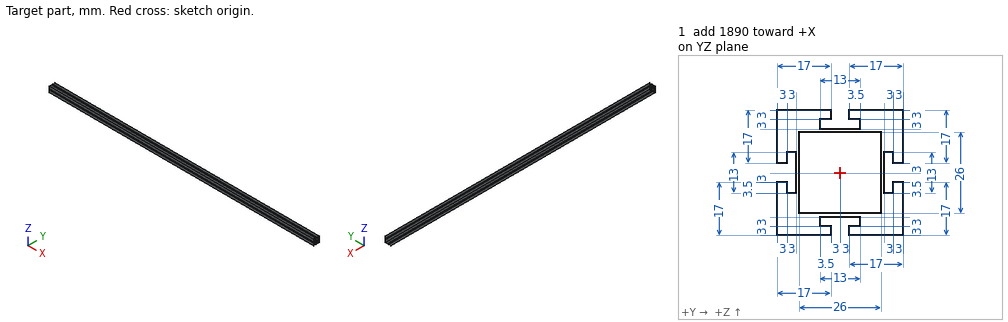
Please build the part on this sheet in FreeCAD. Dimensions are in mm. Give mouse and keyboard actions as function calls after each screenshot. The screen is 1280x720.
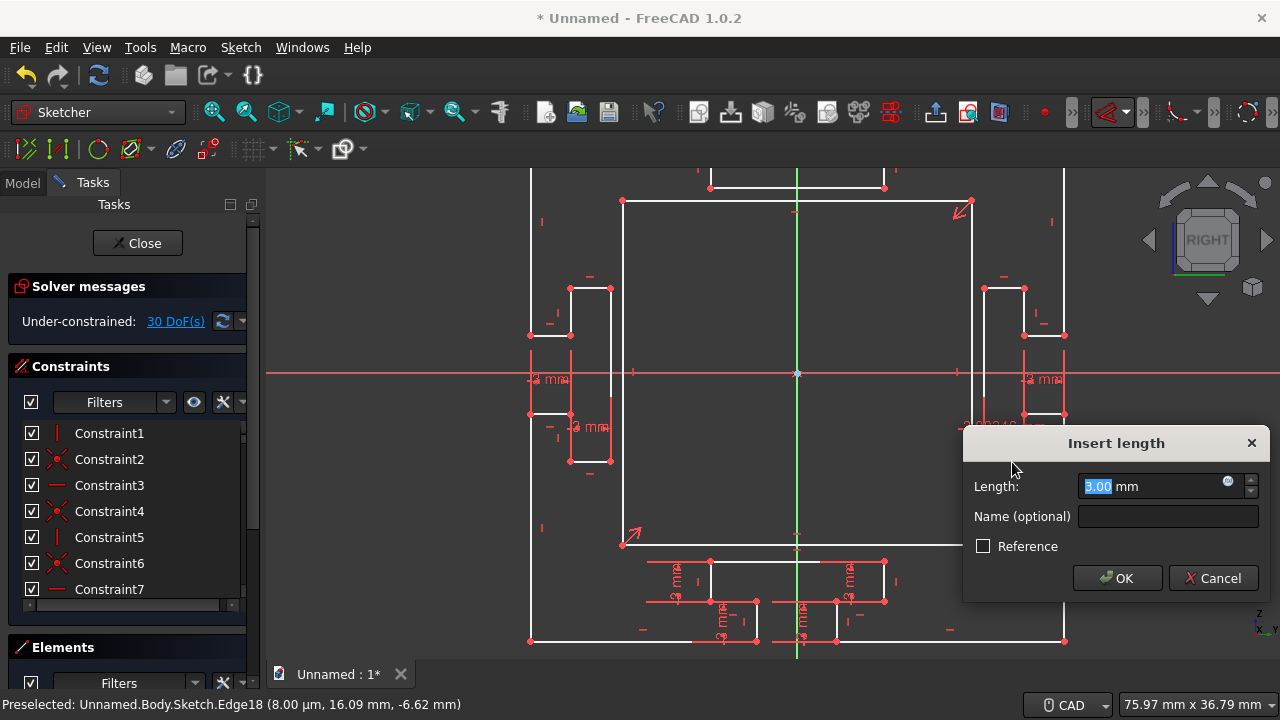
text(3)
key(Return)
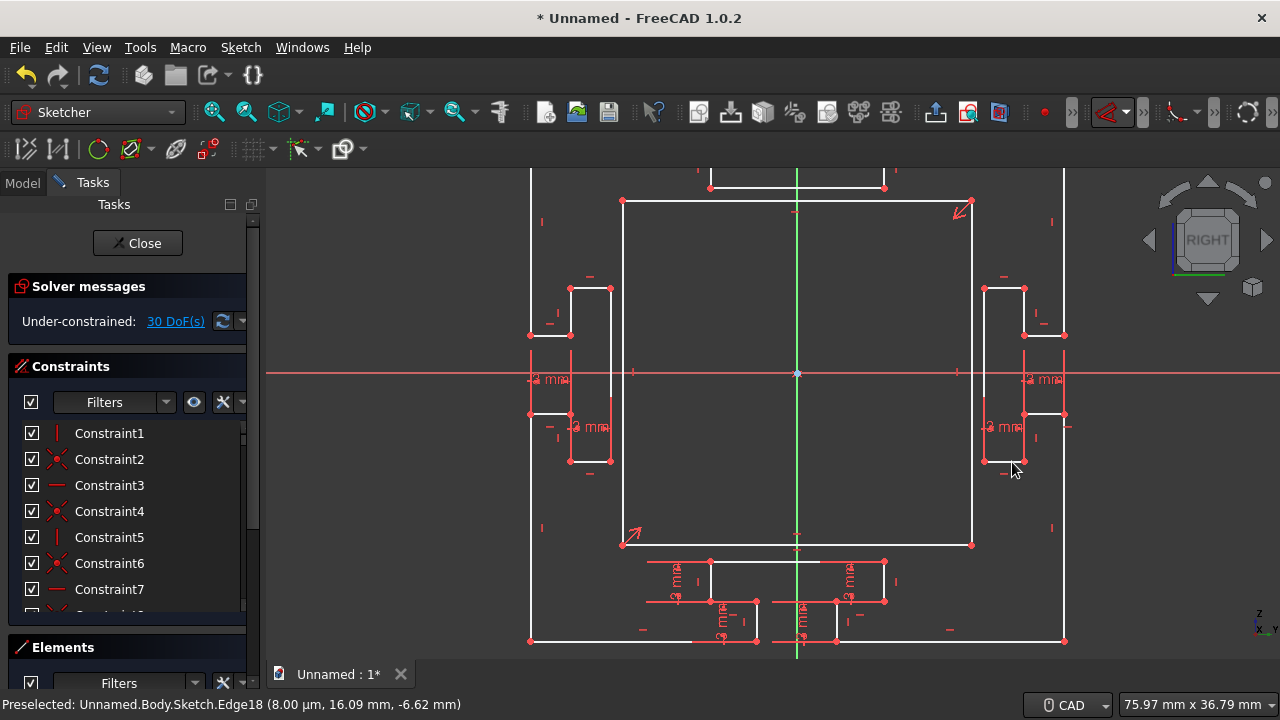
click(996, 288)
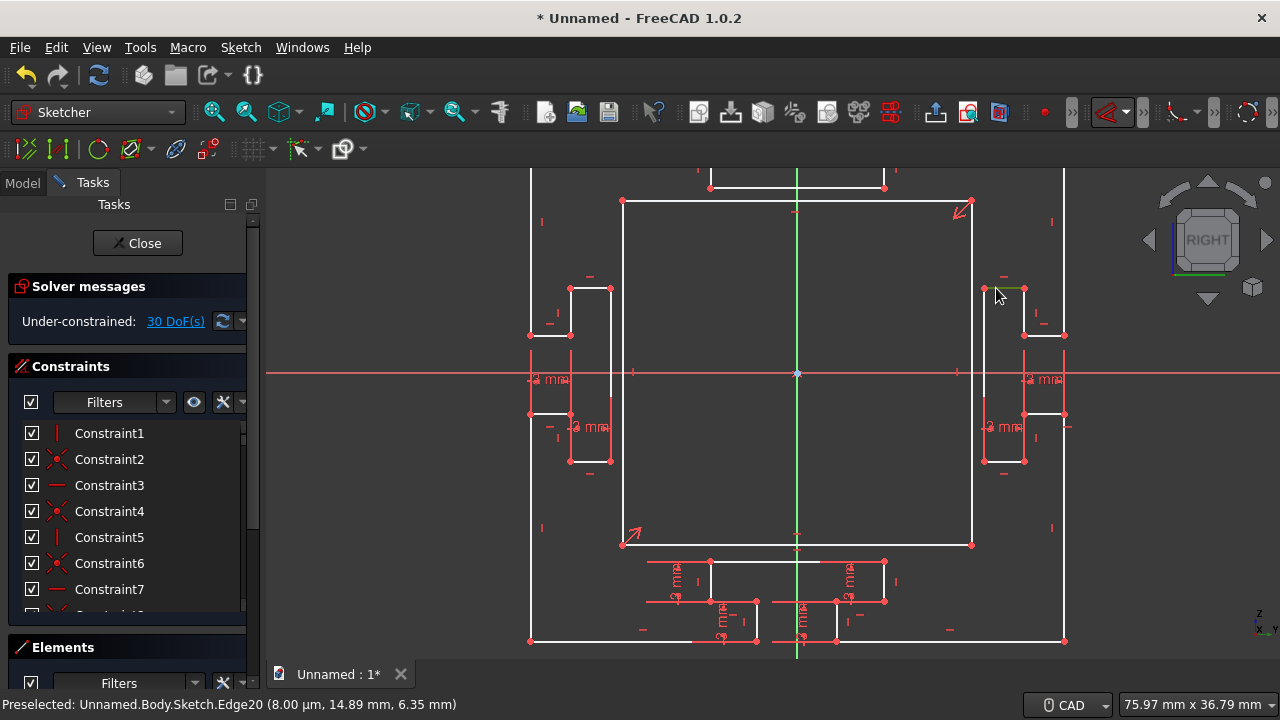
key(l)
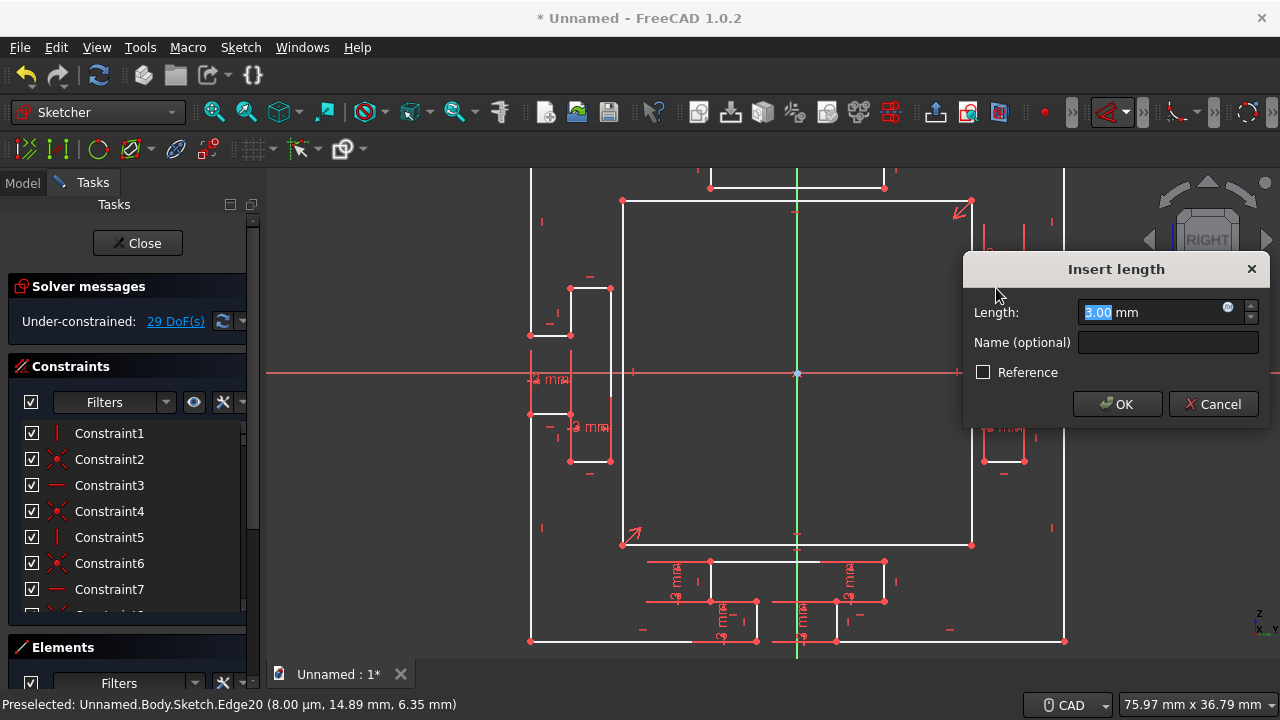
text(3)
key(Return)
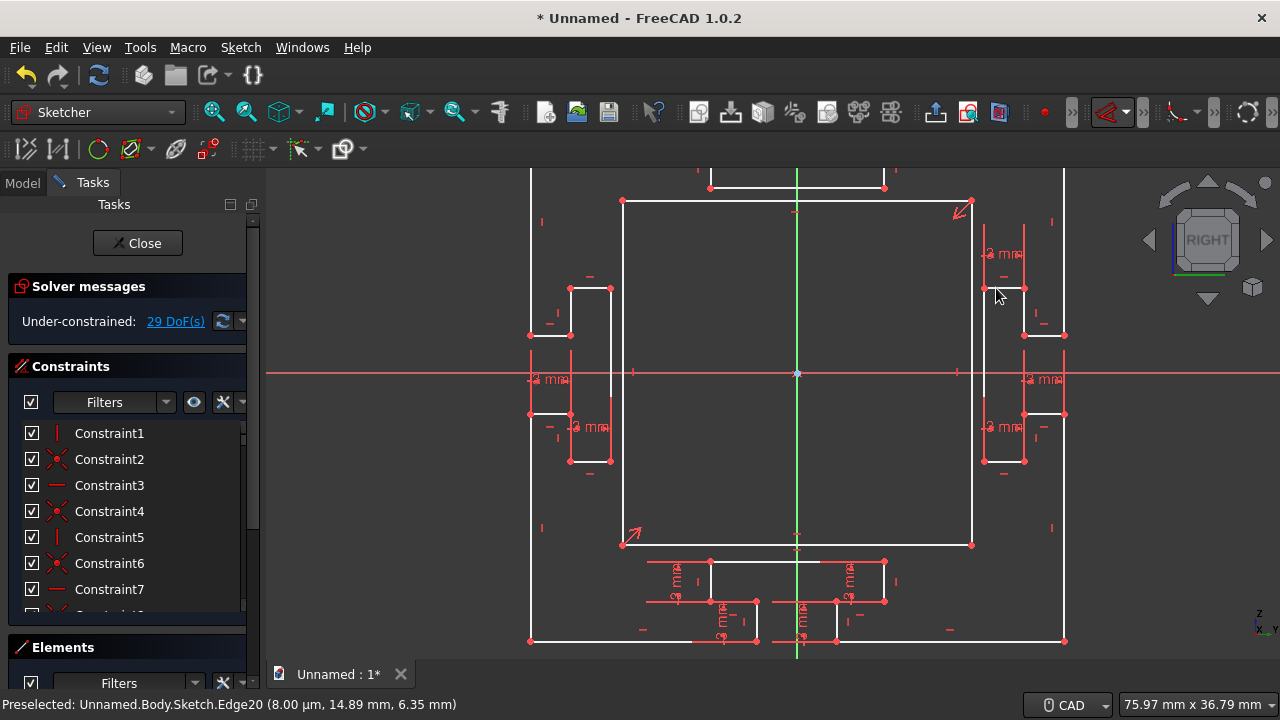
click(1036, 336)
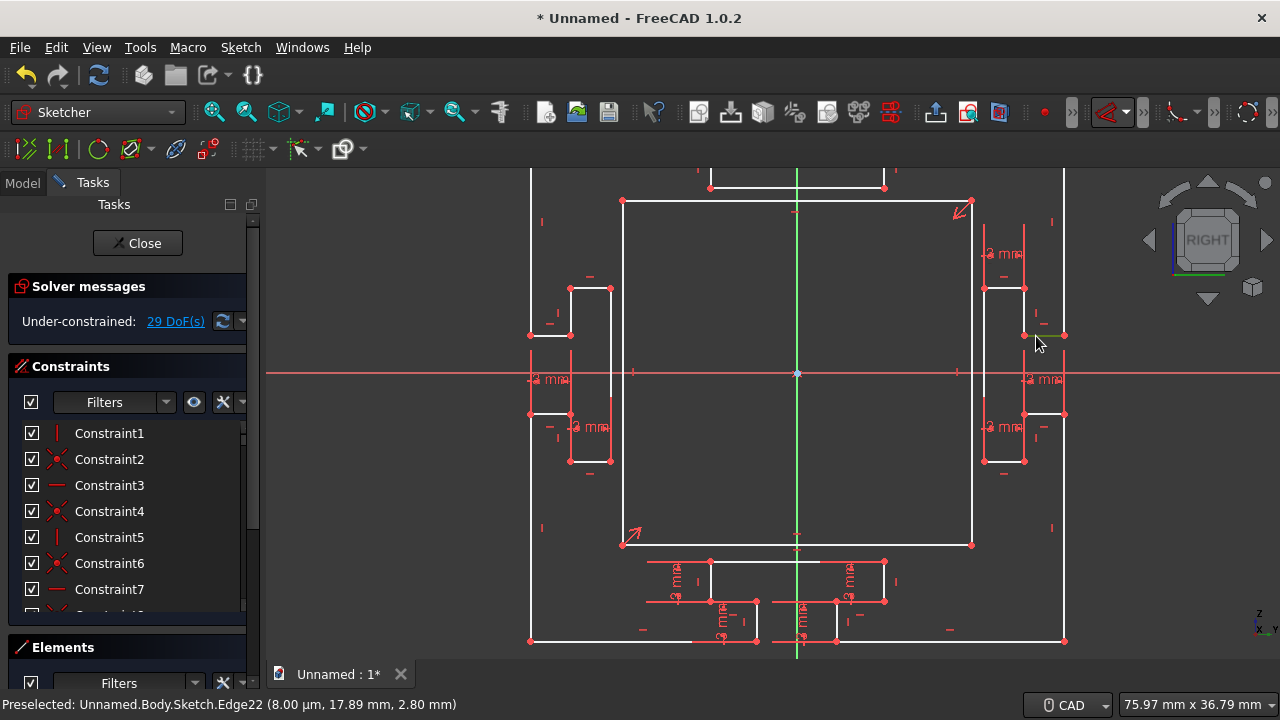
click(1128, 112)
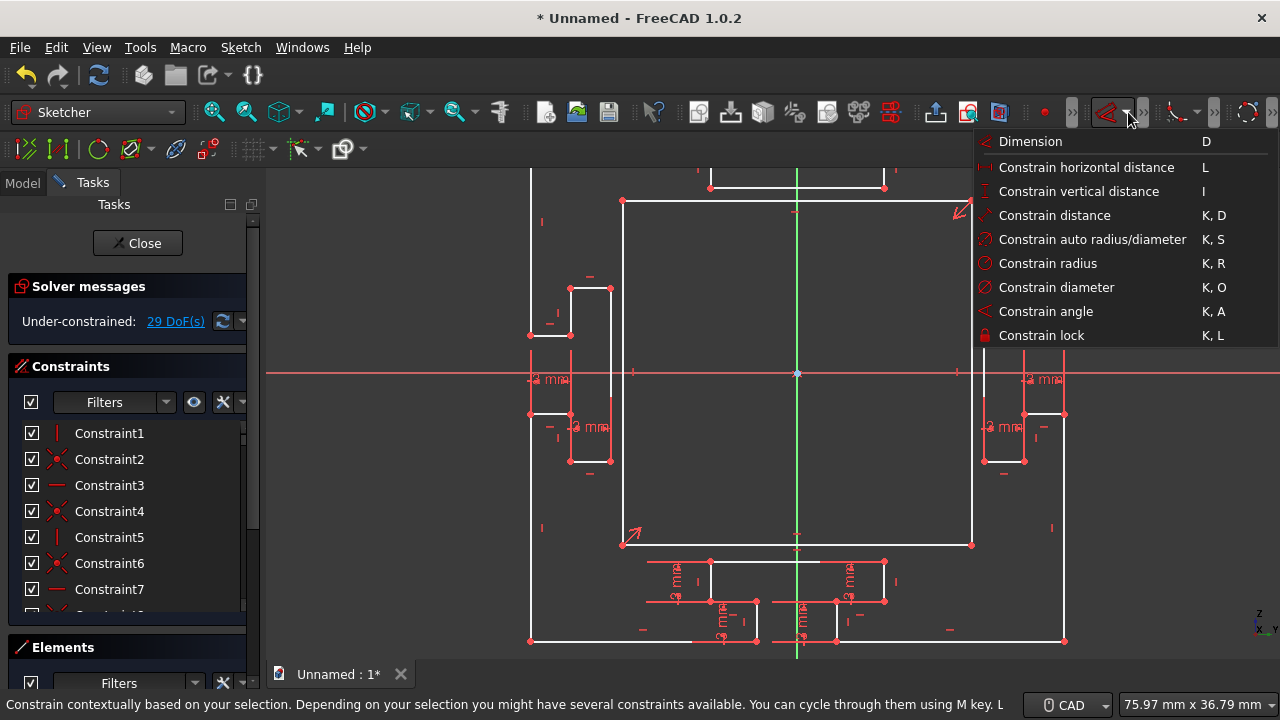
click(1126, 167)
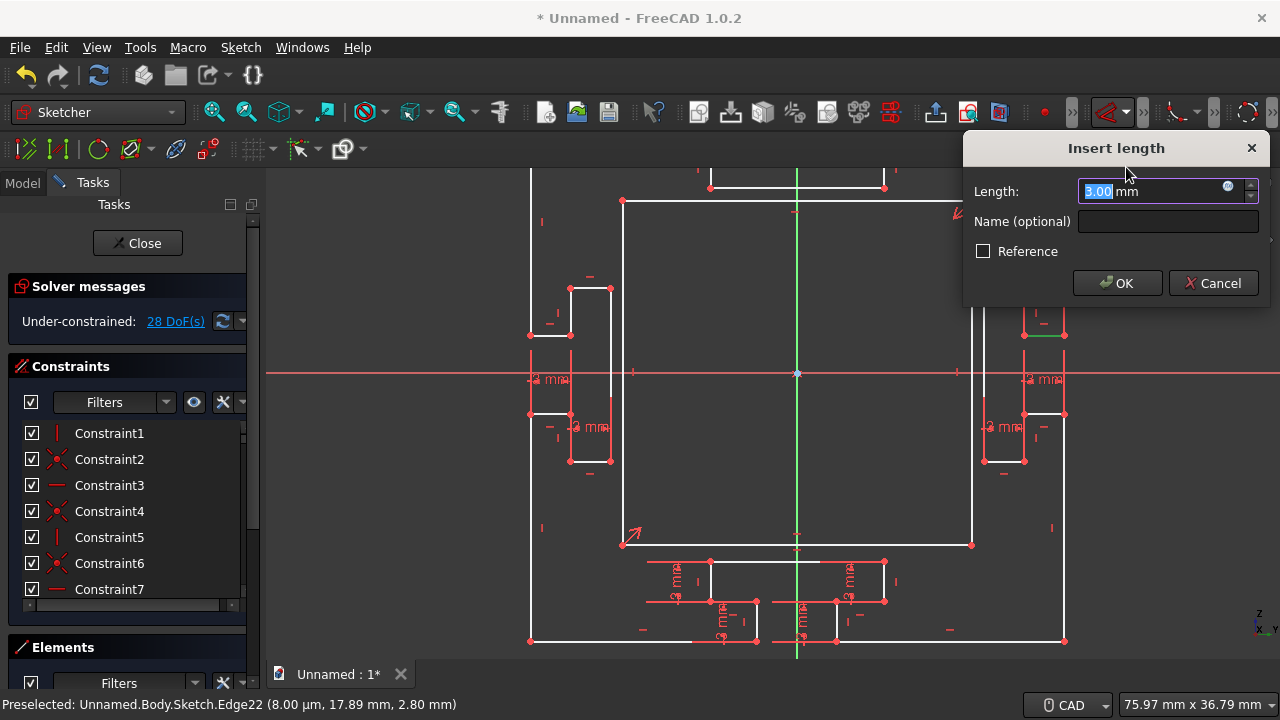
text(3)
key(Return)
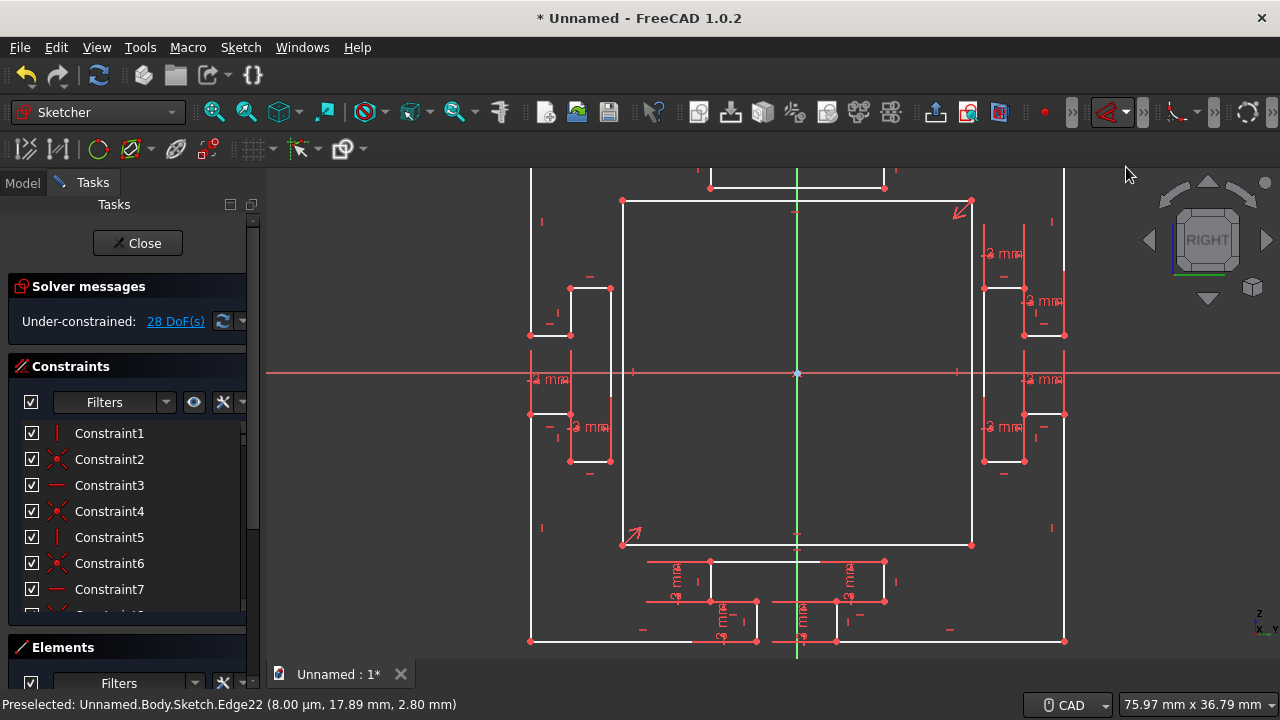
scroll(592, 463, down, 3)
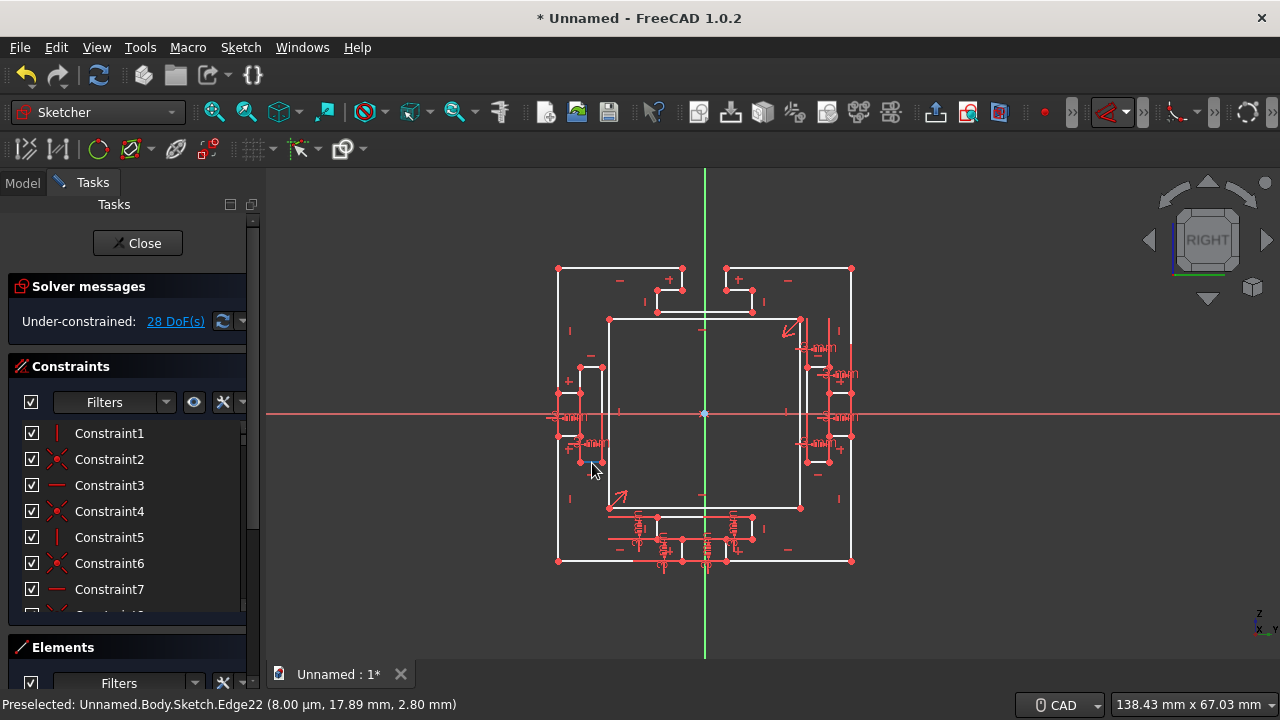
scroll(726, 275, up, 4)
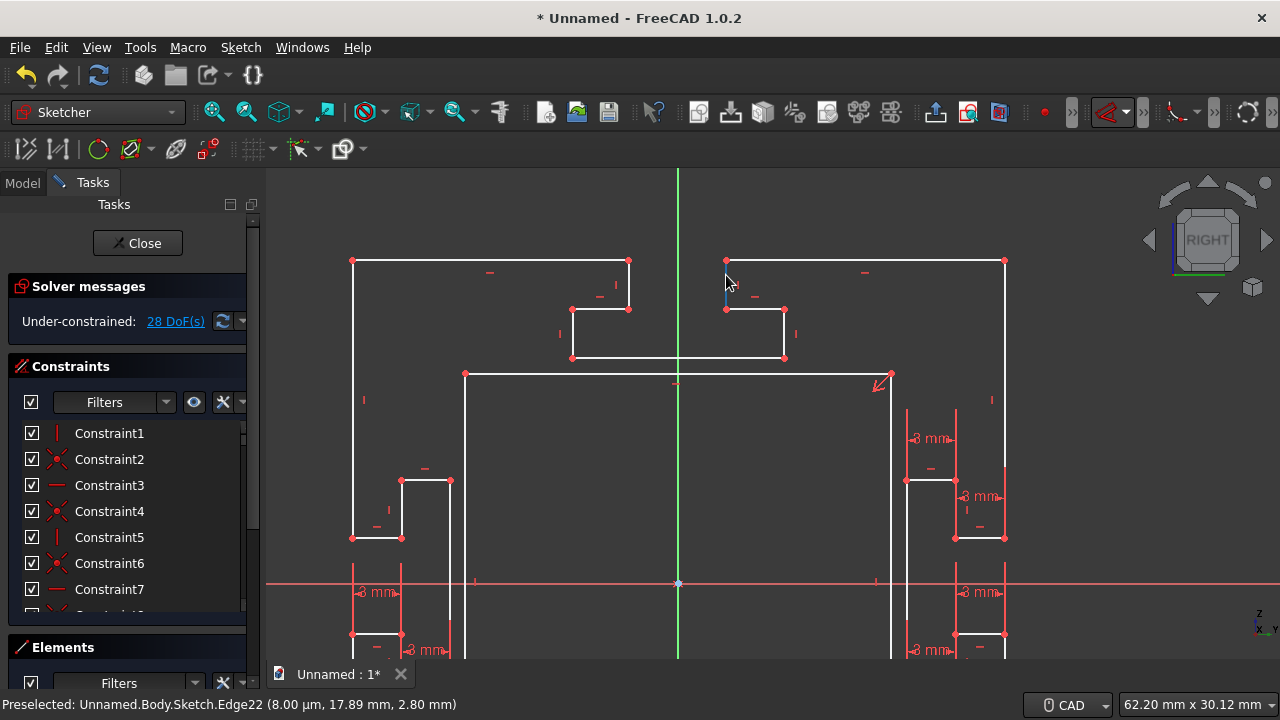
click(726, 275)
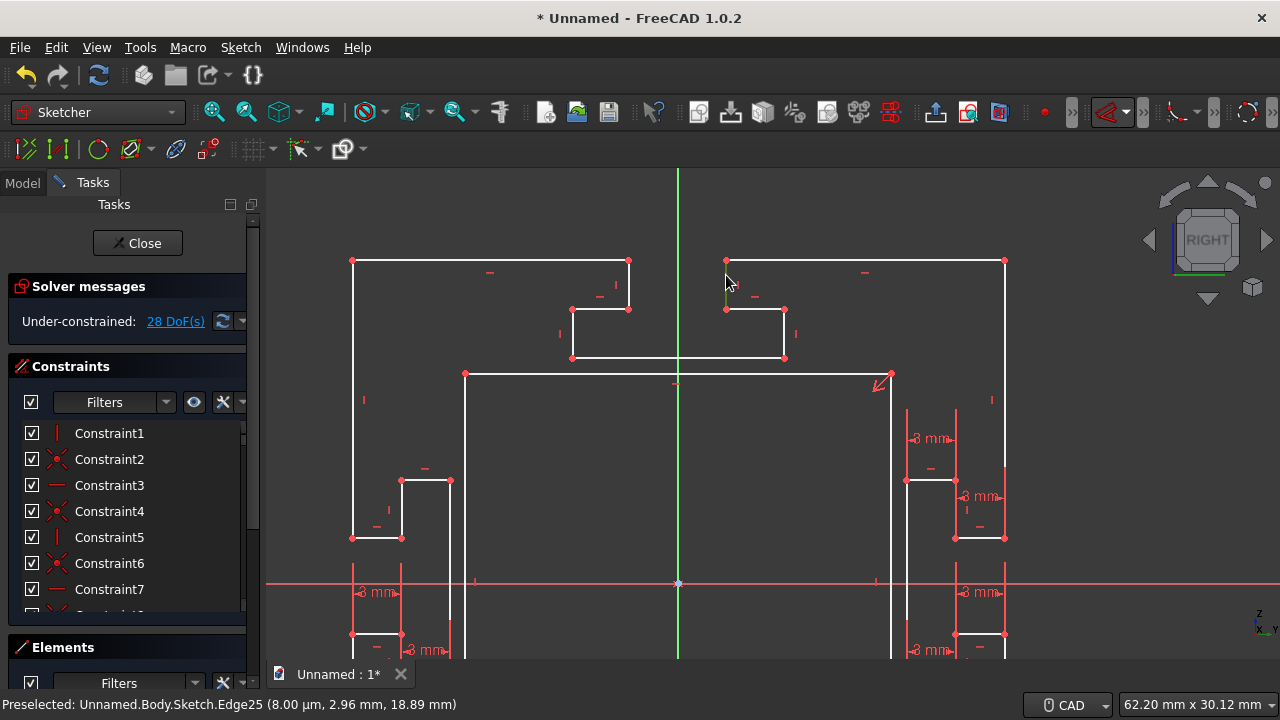
click(1128, 112)